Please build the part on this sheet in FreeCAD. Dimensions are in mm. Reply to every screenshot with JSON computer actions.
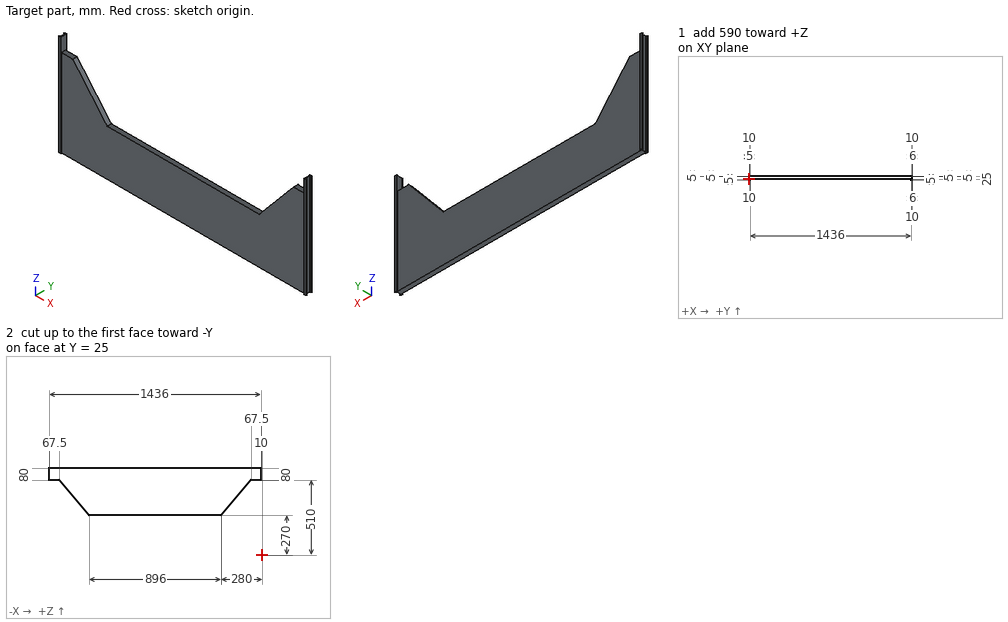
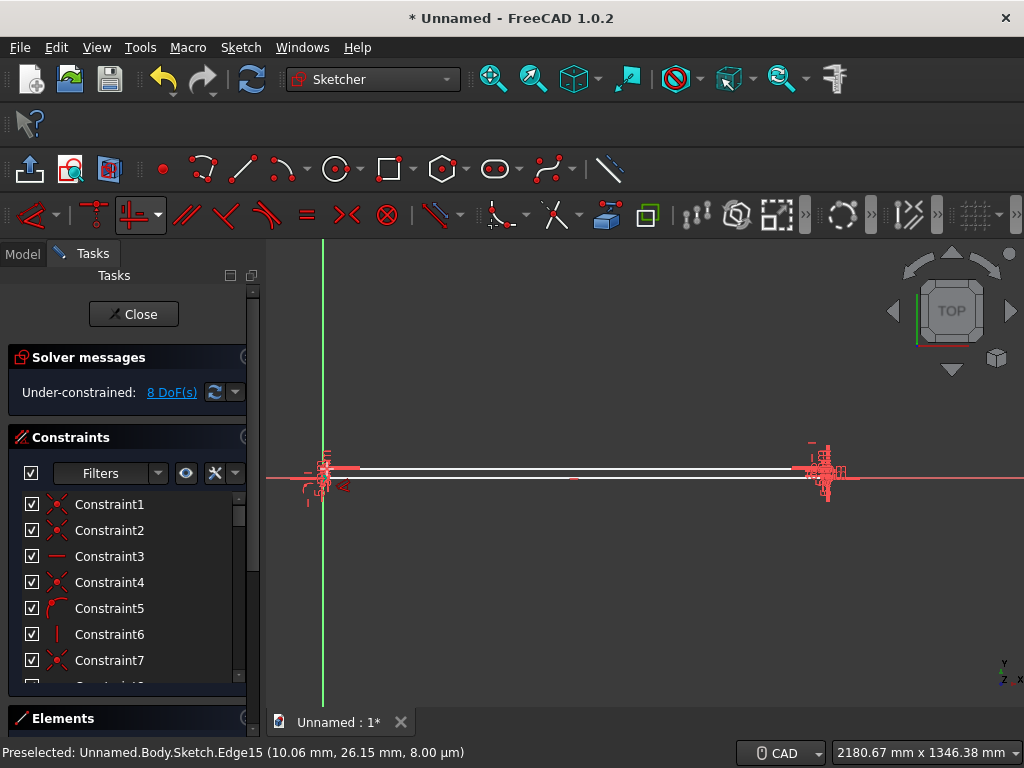
{"action": "scroll", "coordinate": [323, 468], "scroll_direction": "up", "scroll_amount": 16}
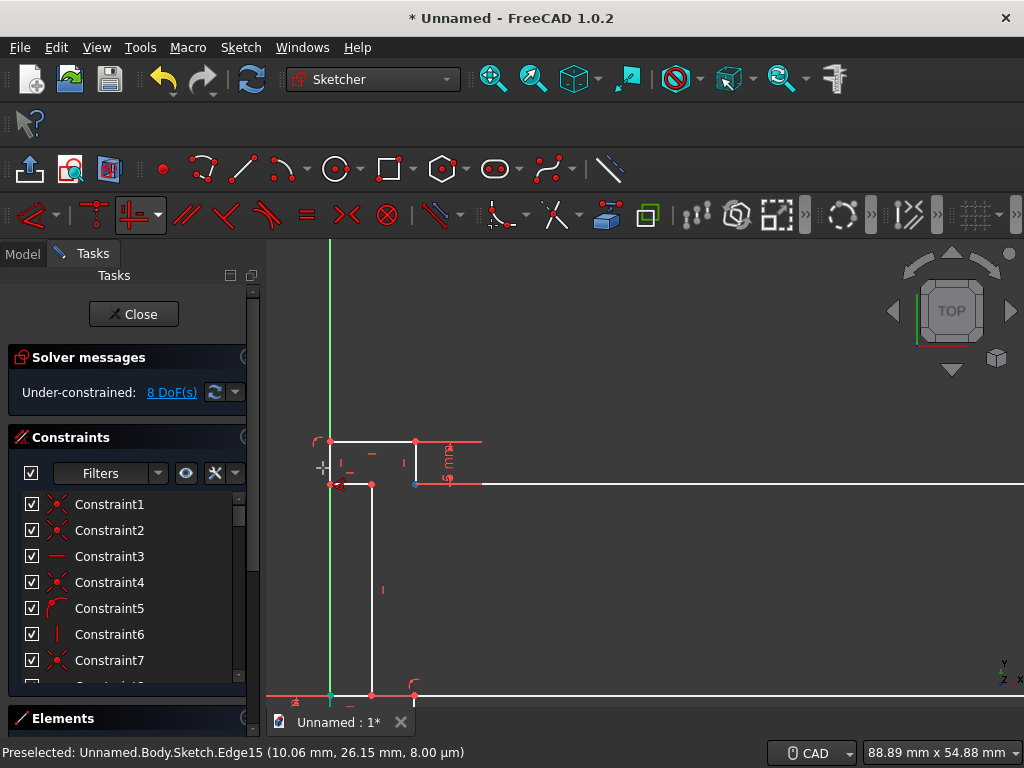
{"action": "left_click", "coordinate": [330, 454]}
{"action": "left_click", "coordinate": [296, 463]}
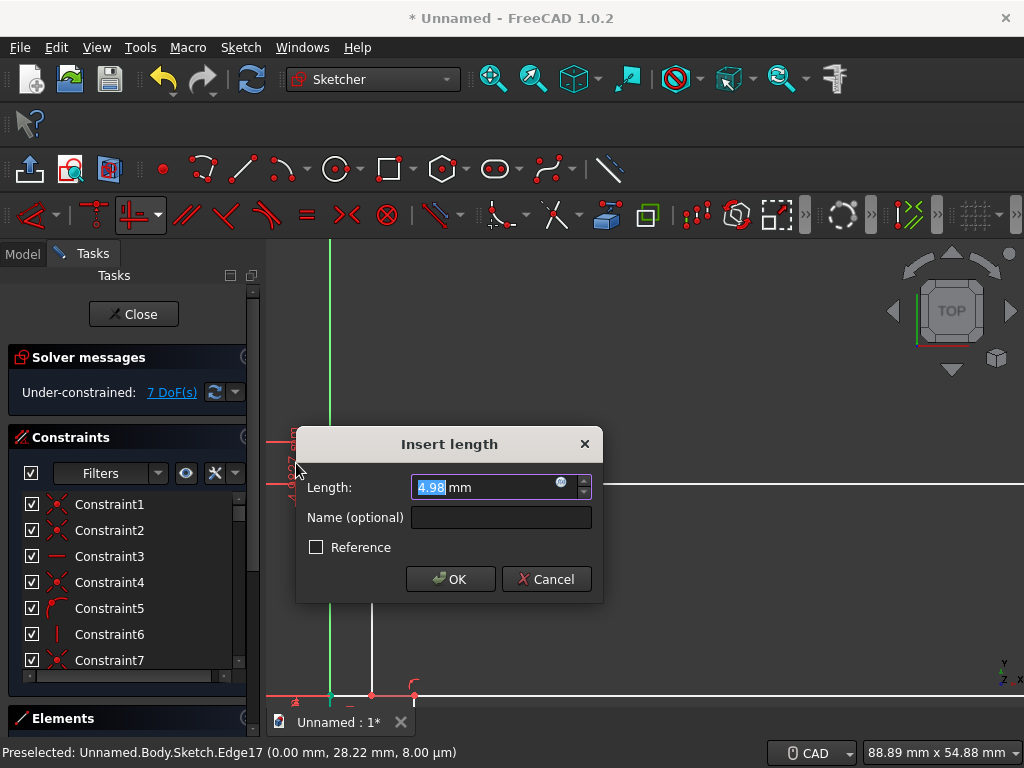
{"action": "type", "text": "5"}
{"action": "key", "text": "Return"}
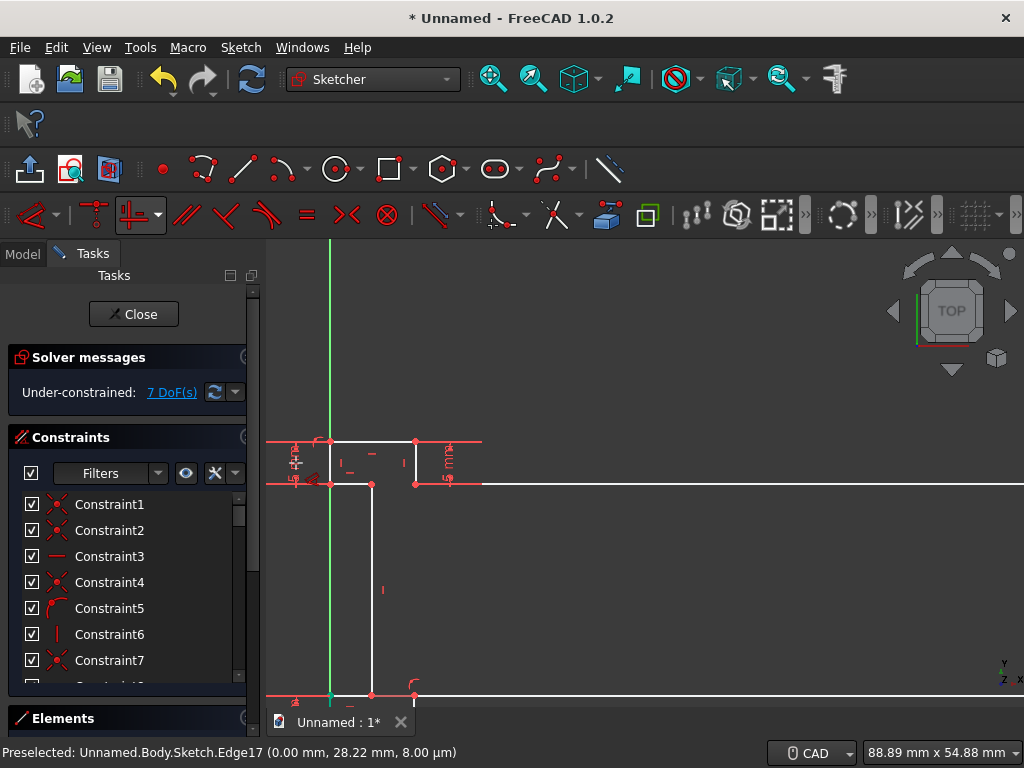
{"action": "left_click", "coordinate": [343, 484]}
{"action": "left_click", "coordinate": [351, 518]}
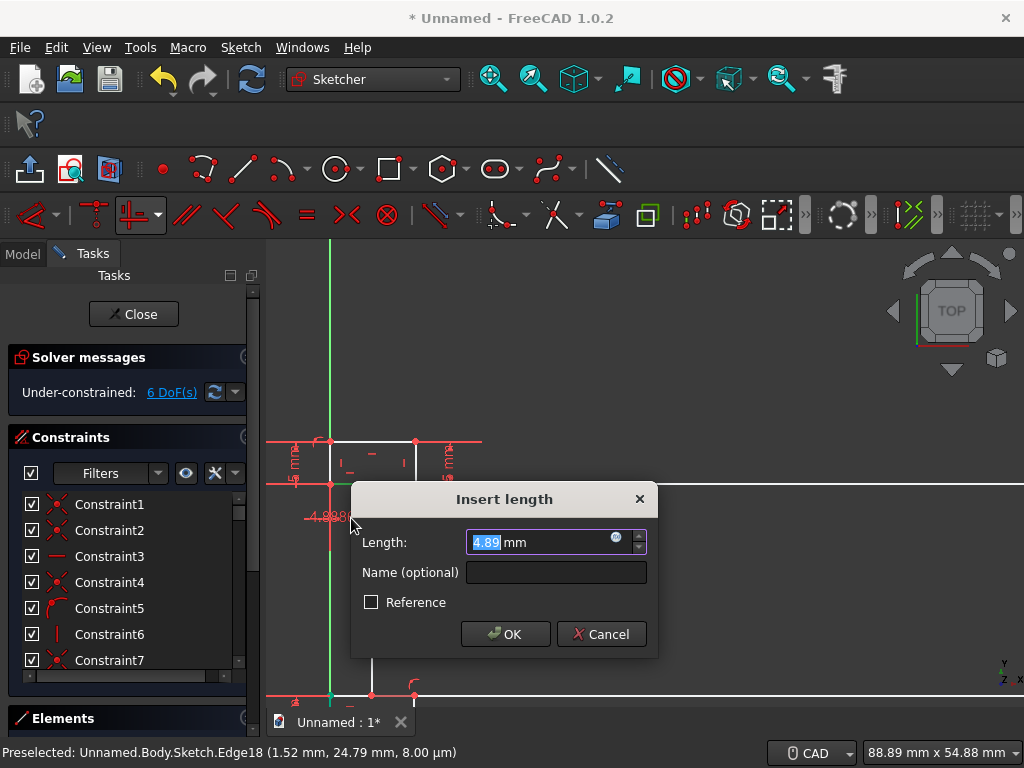
{"action": "type", "text": "5"}
{"action": "key", "text": "Return"}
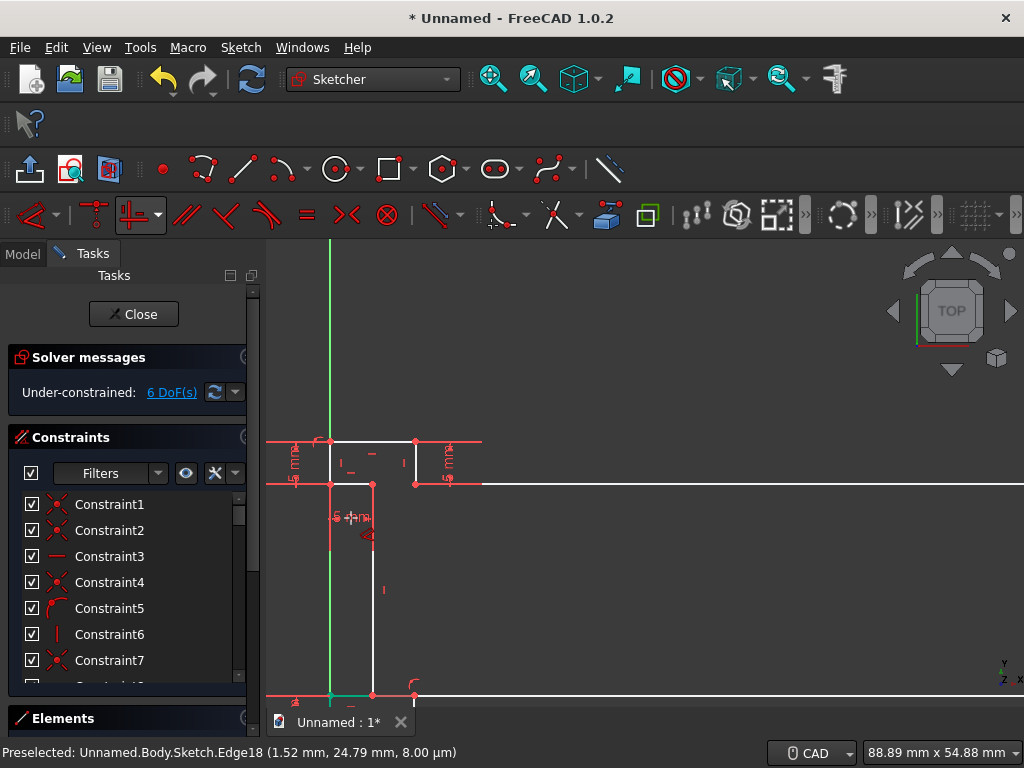
{"action": "scroll", "coordinate": [323, 468], "scroll_direction": "down", "scroll_amount": 16}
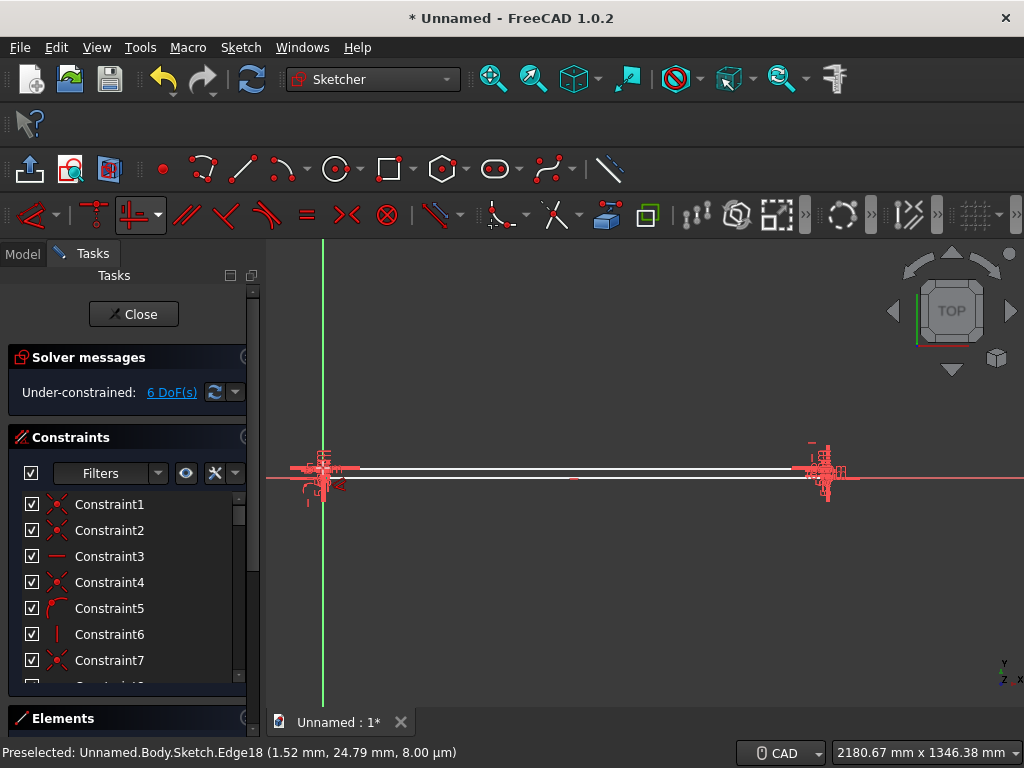
{"action": "scroll", "coordinate": [324, 479], "scroll_direction": "up", "scroll_amount": 13}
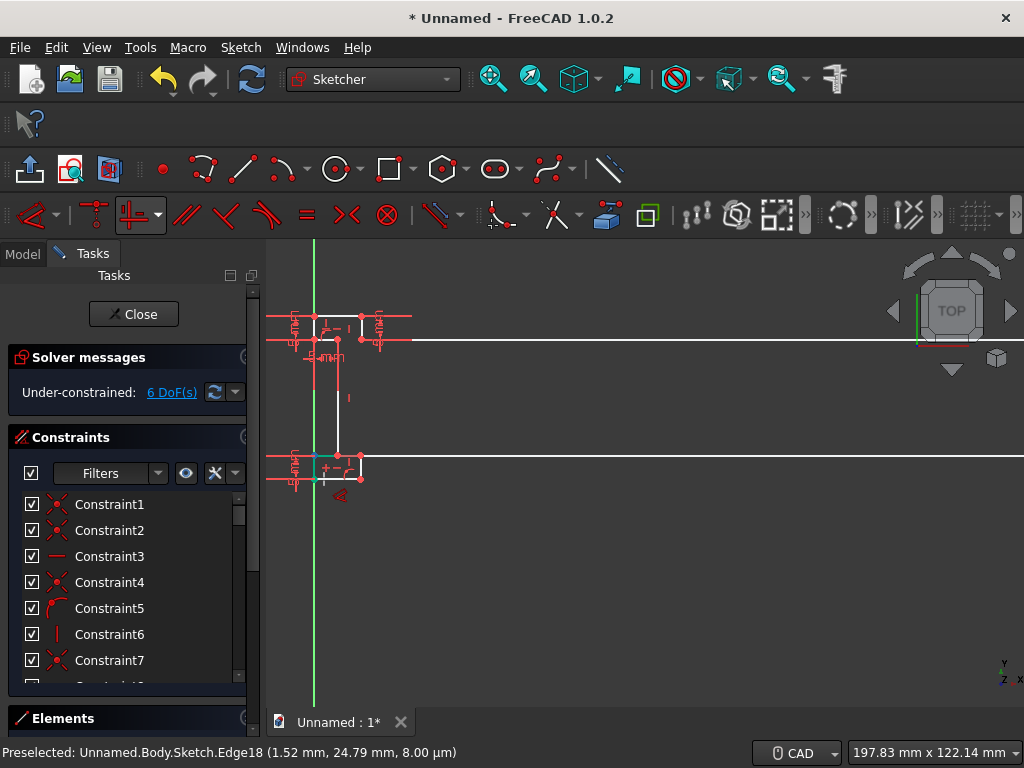
{"action": "left_click", "coordinate": [328, 479]}
{"action": "left_click", "coordinate": [338, 513]}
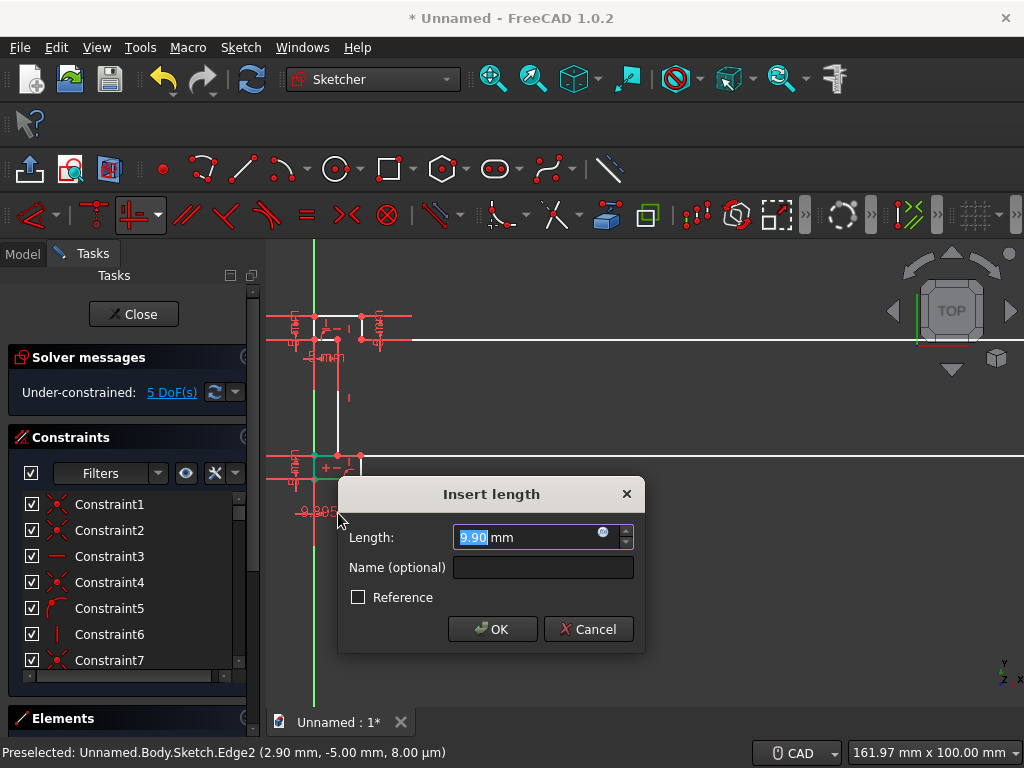
{"action": "type", "text": "10"}
{"action": "key", "text": "Return"}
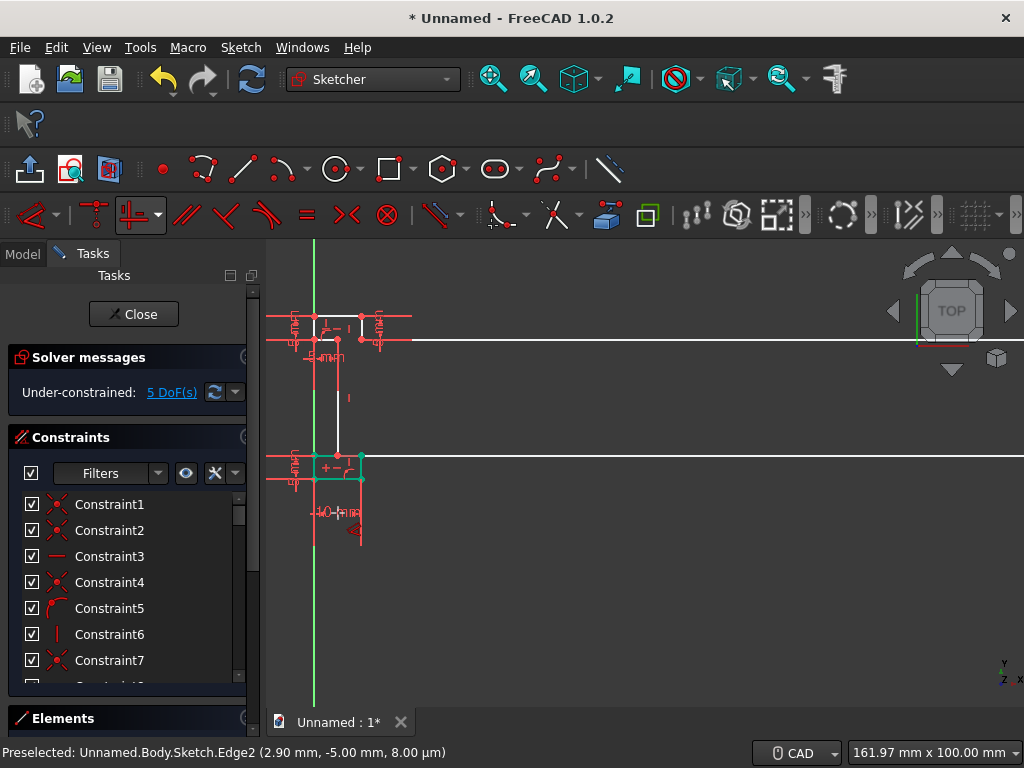
{"action": "scroll", "coordinate": [373, 478], "scroll_direction": "down", "scroll_amount": 14}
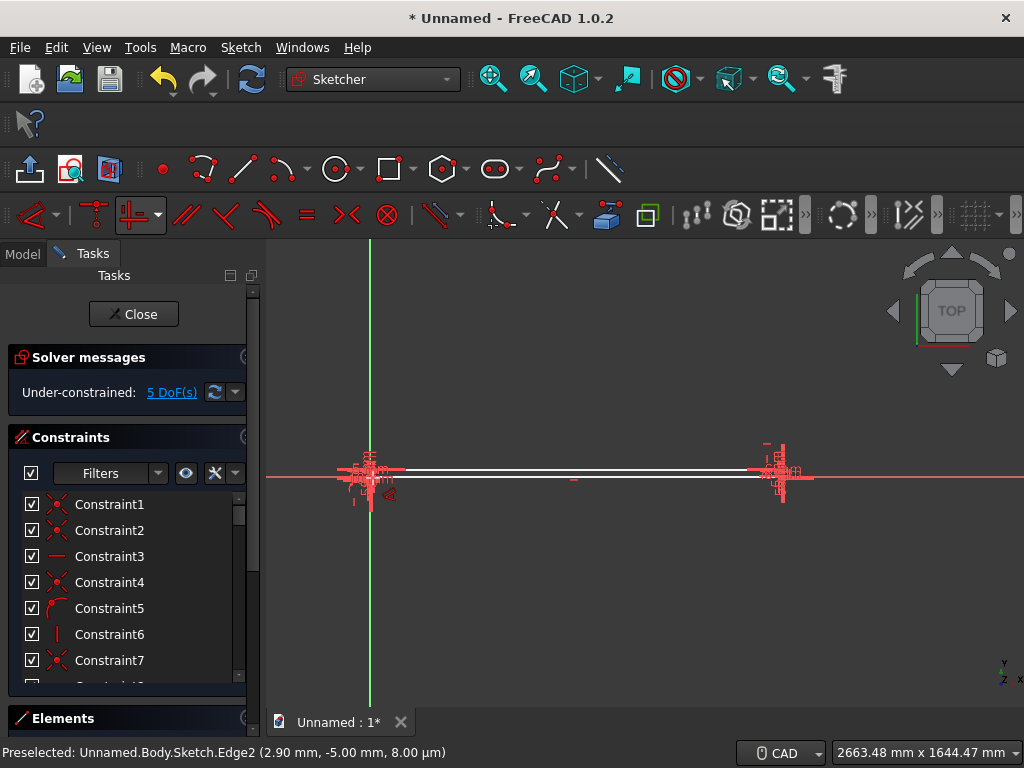
{"action": "scroll", "coordinate": [782, 479], "scroll_direction": "up", "scroll_amount": 14}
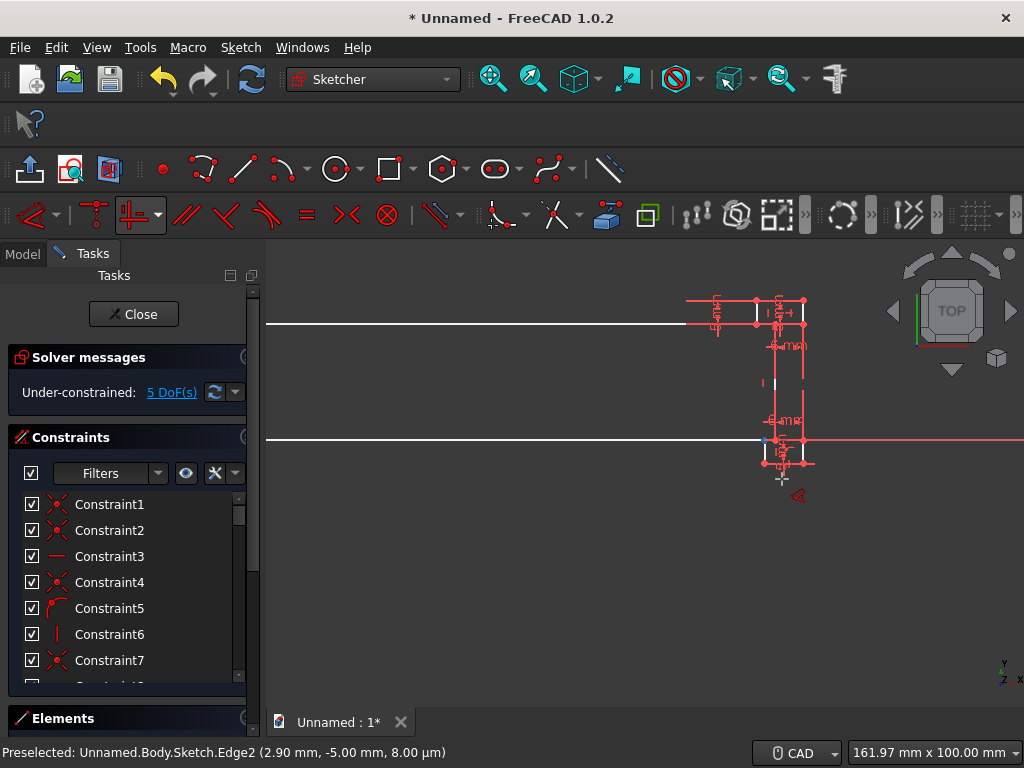
{"action": "left_click", "coordinate": [776, 464]}
{"action": "left_click", "coordinate": [784, 498]}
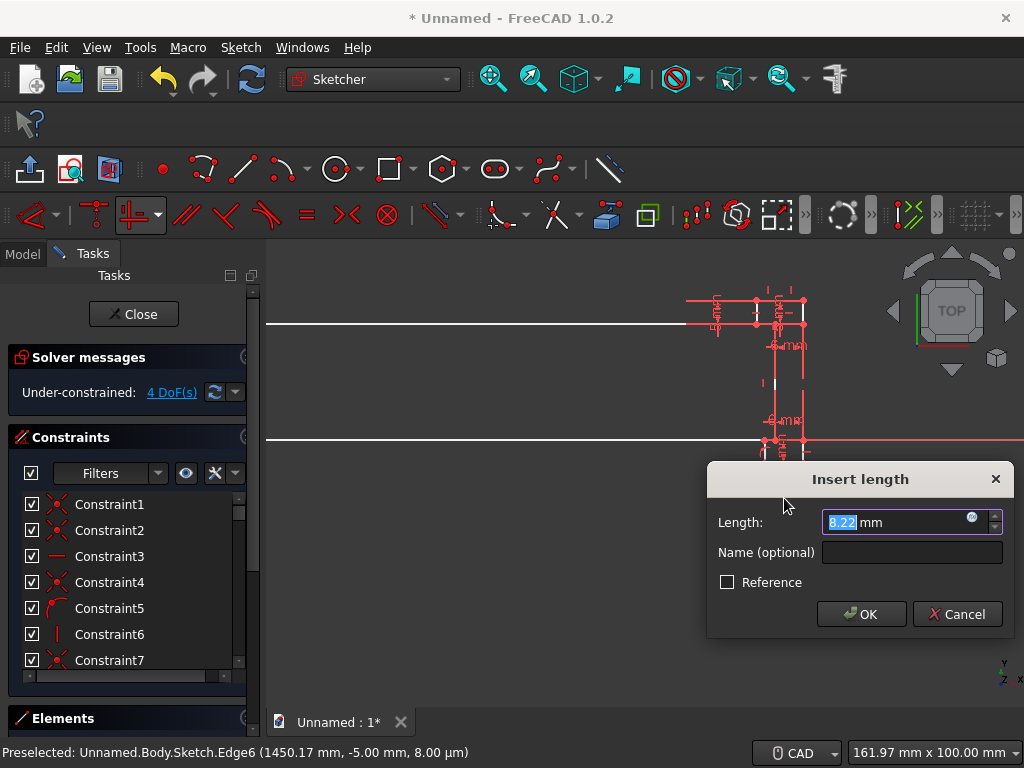
{"action": "type", "text": "10"}
{"action": "key", "text": "Return"}